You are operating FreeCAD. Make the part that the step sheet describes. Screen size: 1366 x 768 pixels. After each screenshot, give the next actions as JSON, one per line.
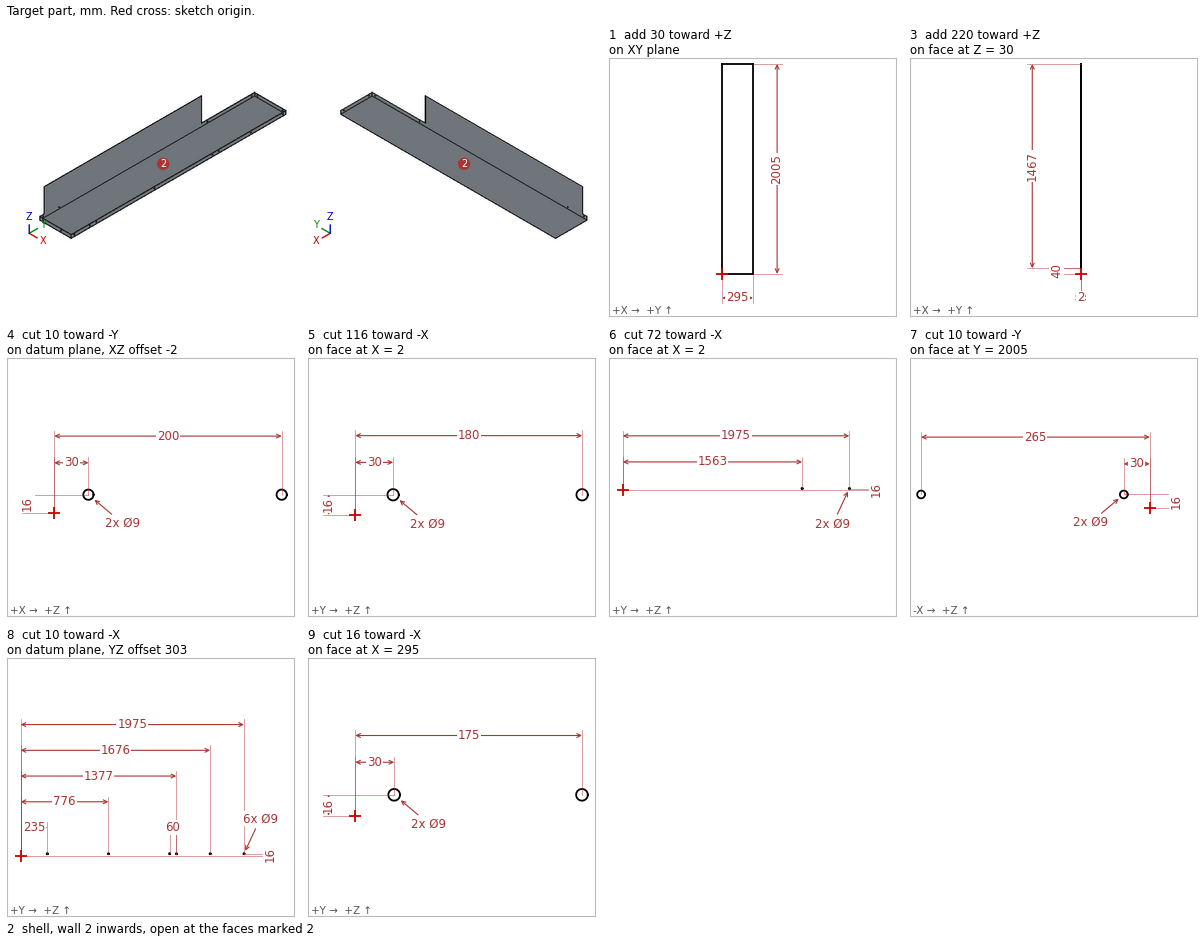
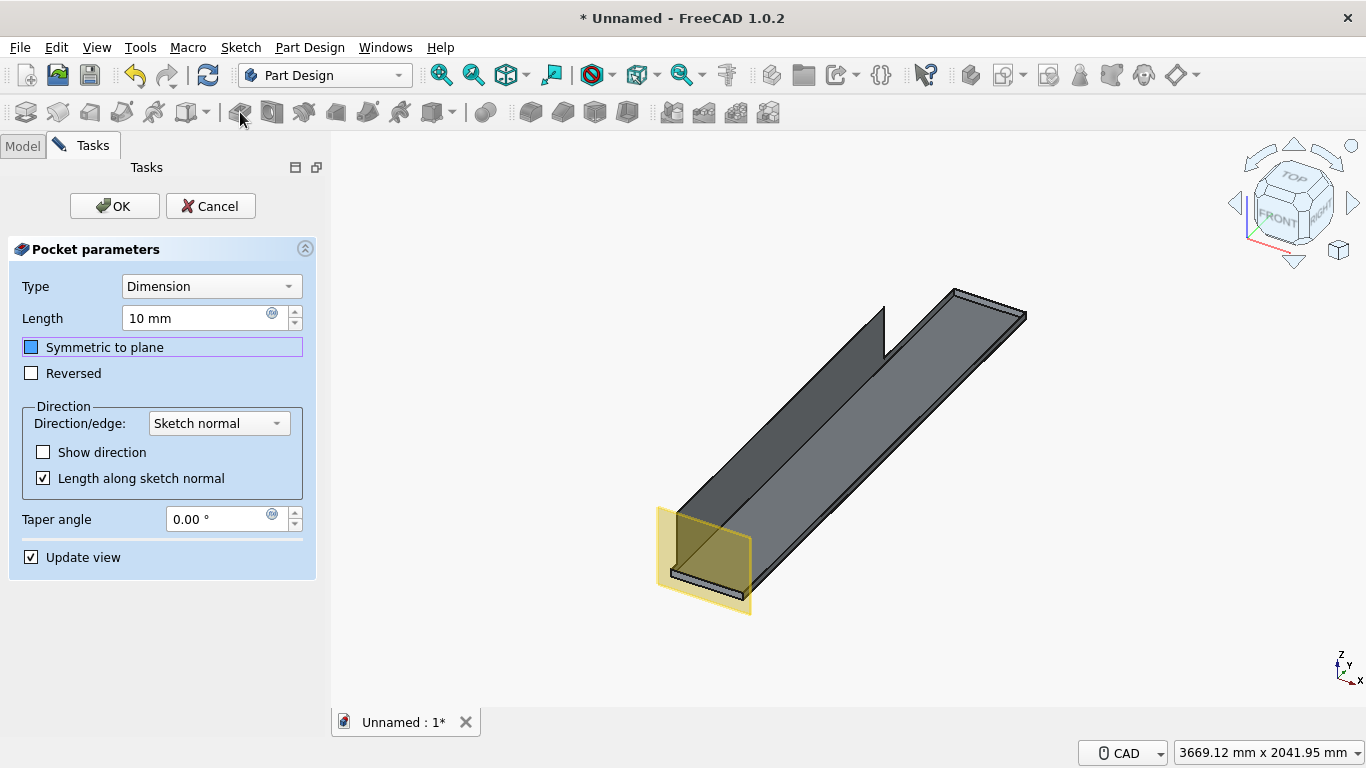
{"action": "left_click", "coordinate": [30, 373]}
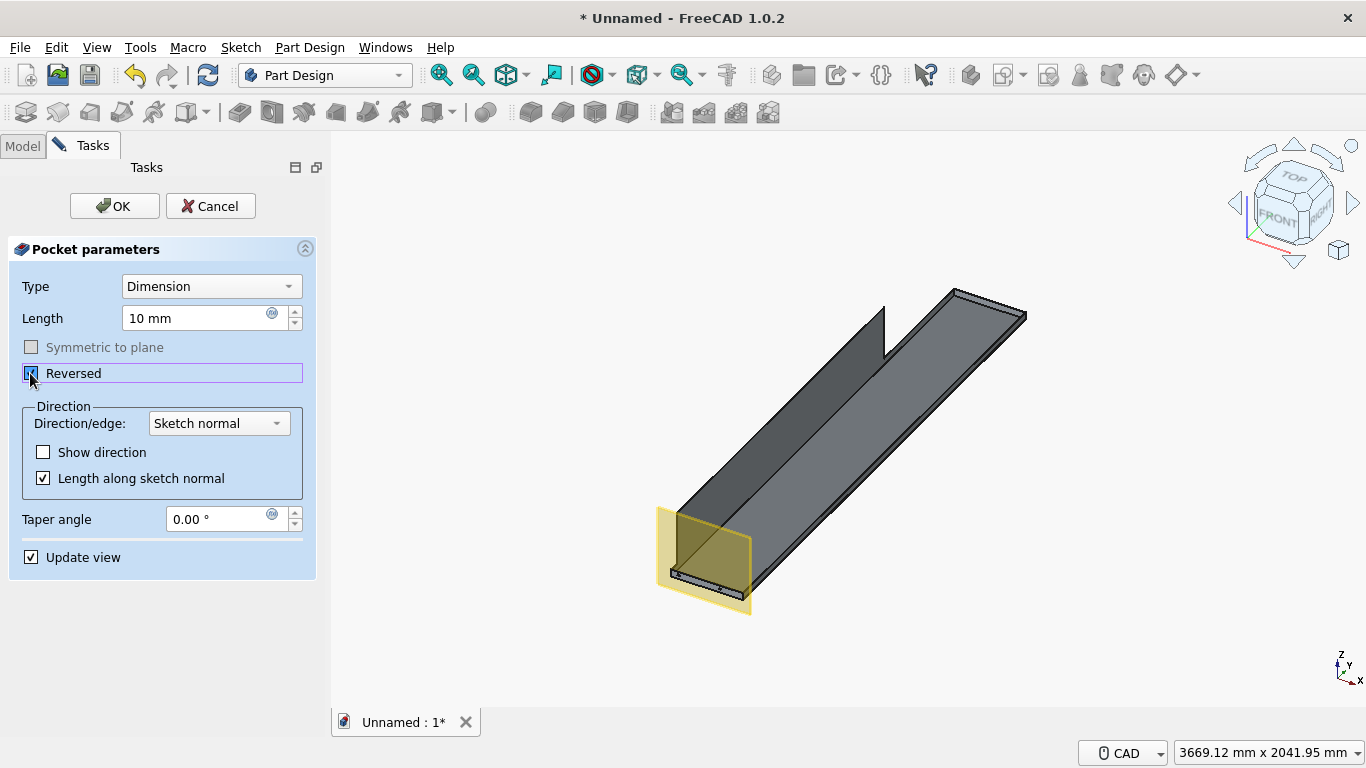
{"action": "left_click", "coordinate": [115, 206]}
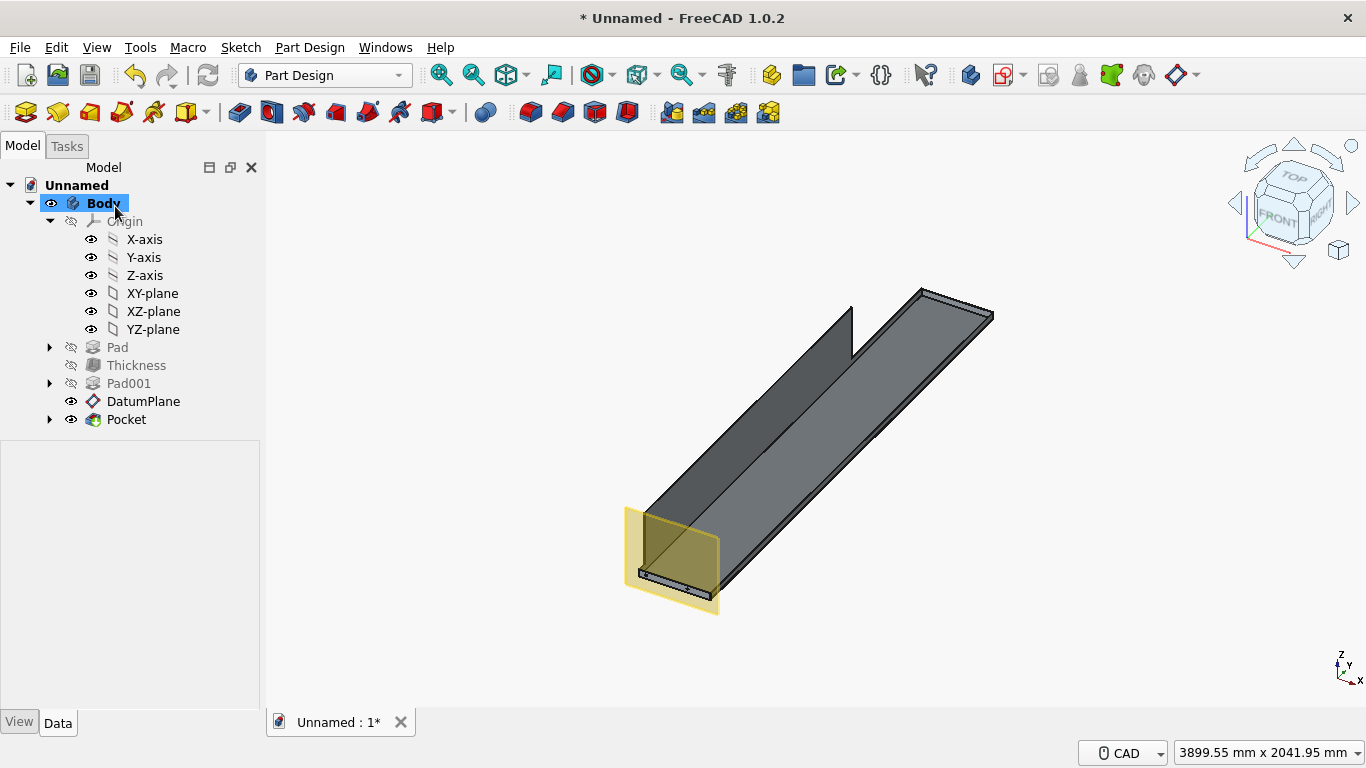
{"action": "left_click", "coordinate": [116, 401]}
{"action": "key", "text": "space"}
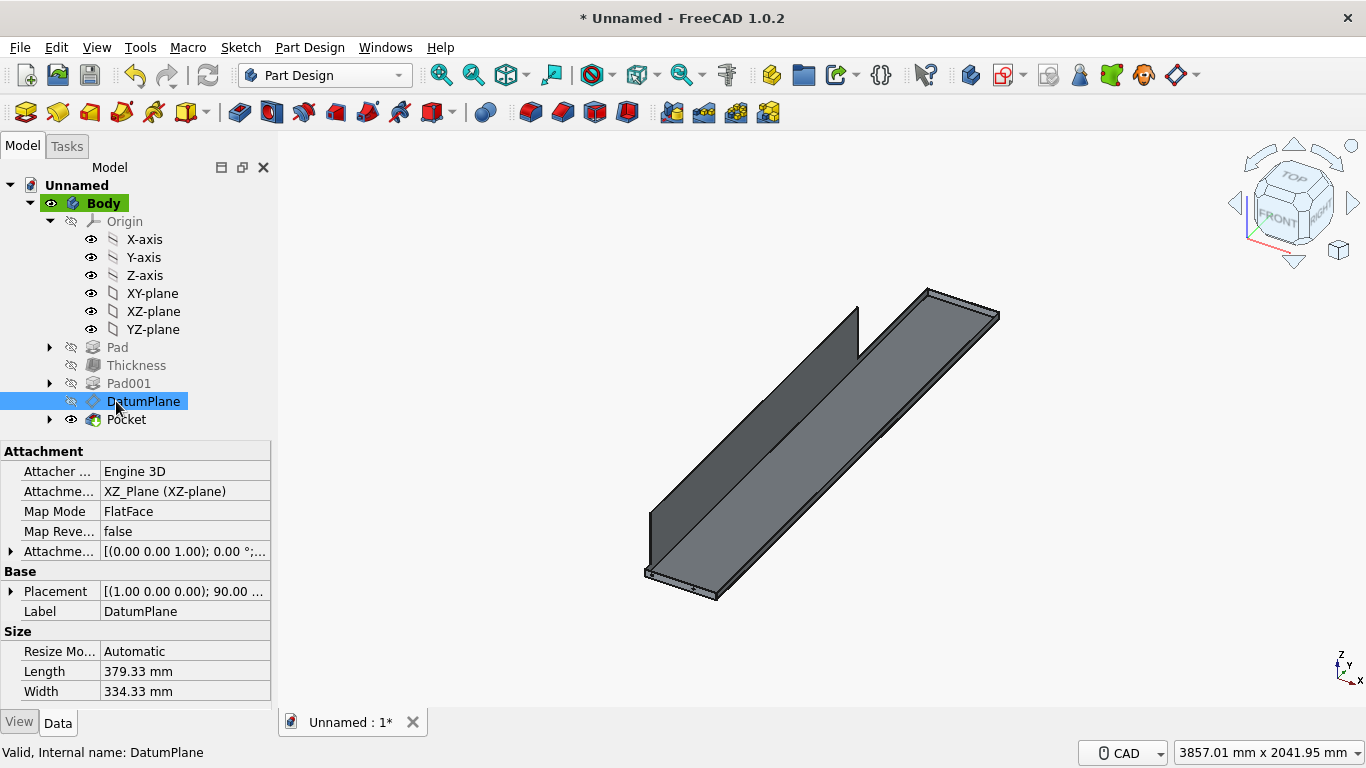
{"action": "left_click", "coordinate": [827, 366]}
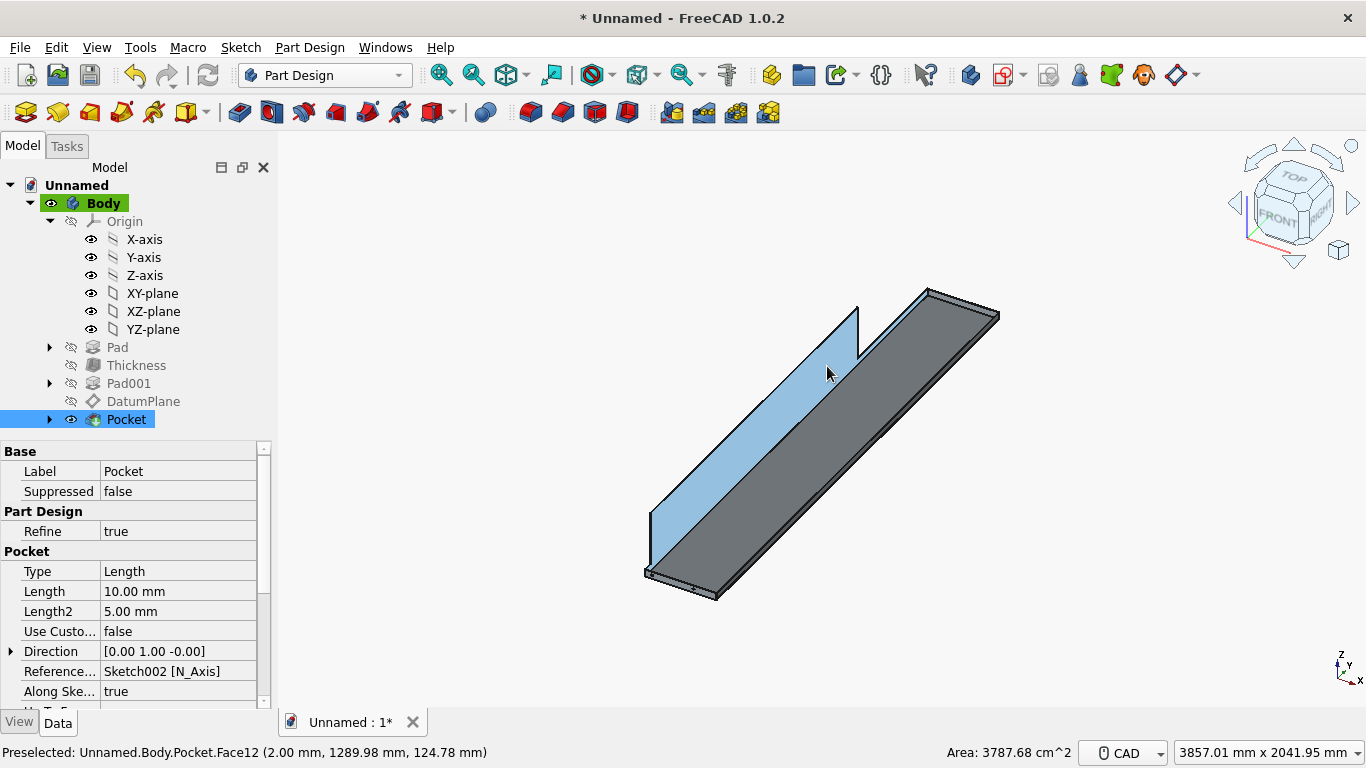
{"action": "left_click", "coordinate": [1004, 76]}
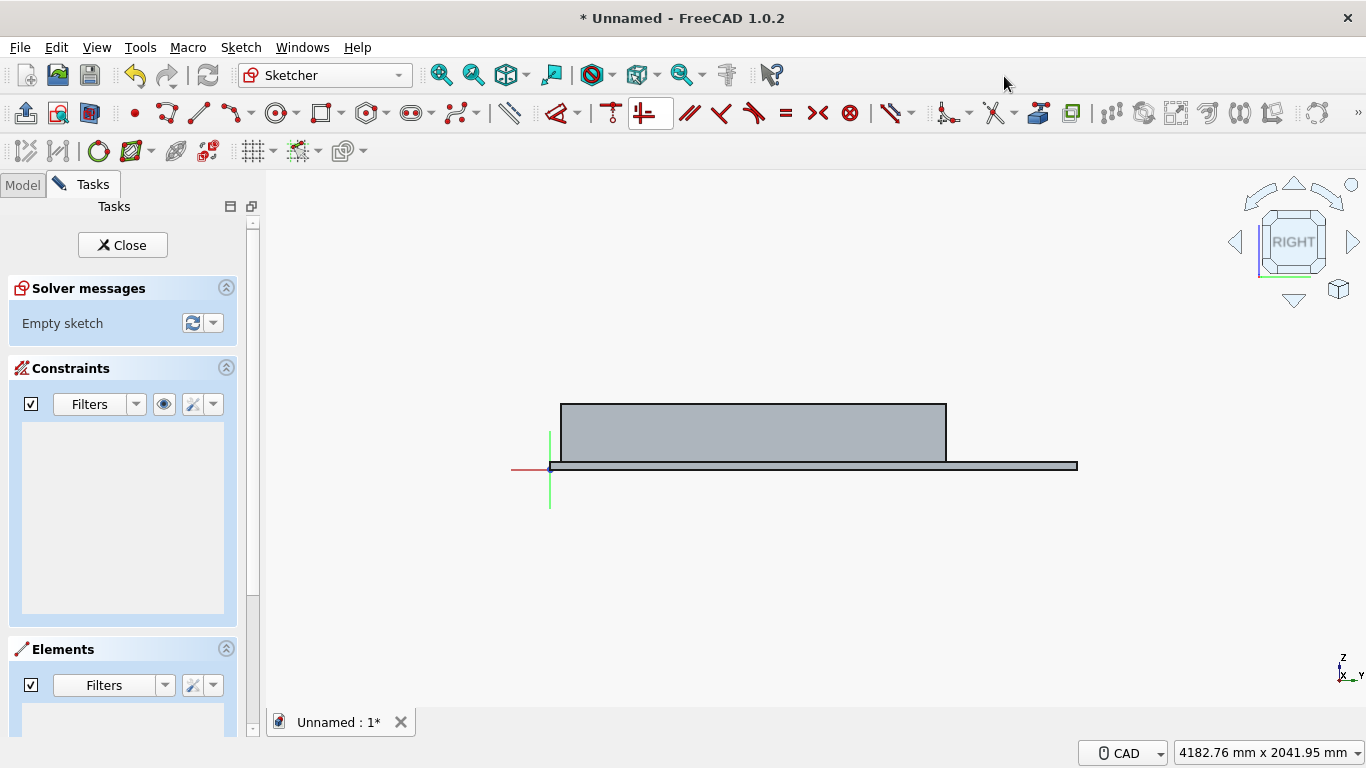
{"action": "scroll", "coordinate": [560, 469], "scroll_direction": "up", "scroll_amount": 13}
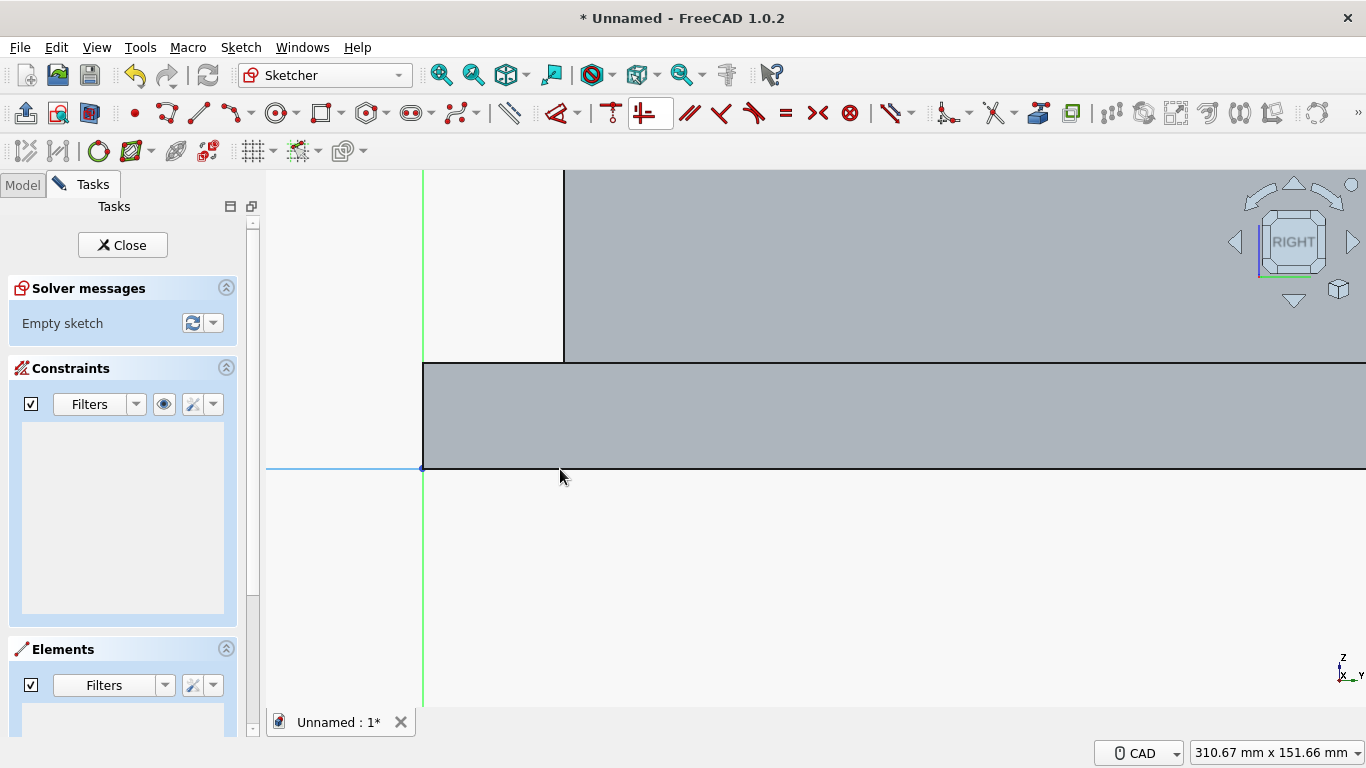
{"action": "key", "text": "g c"}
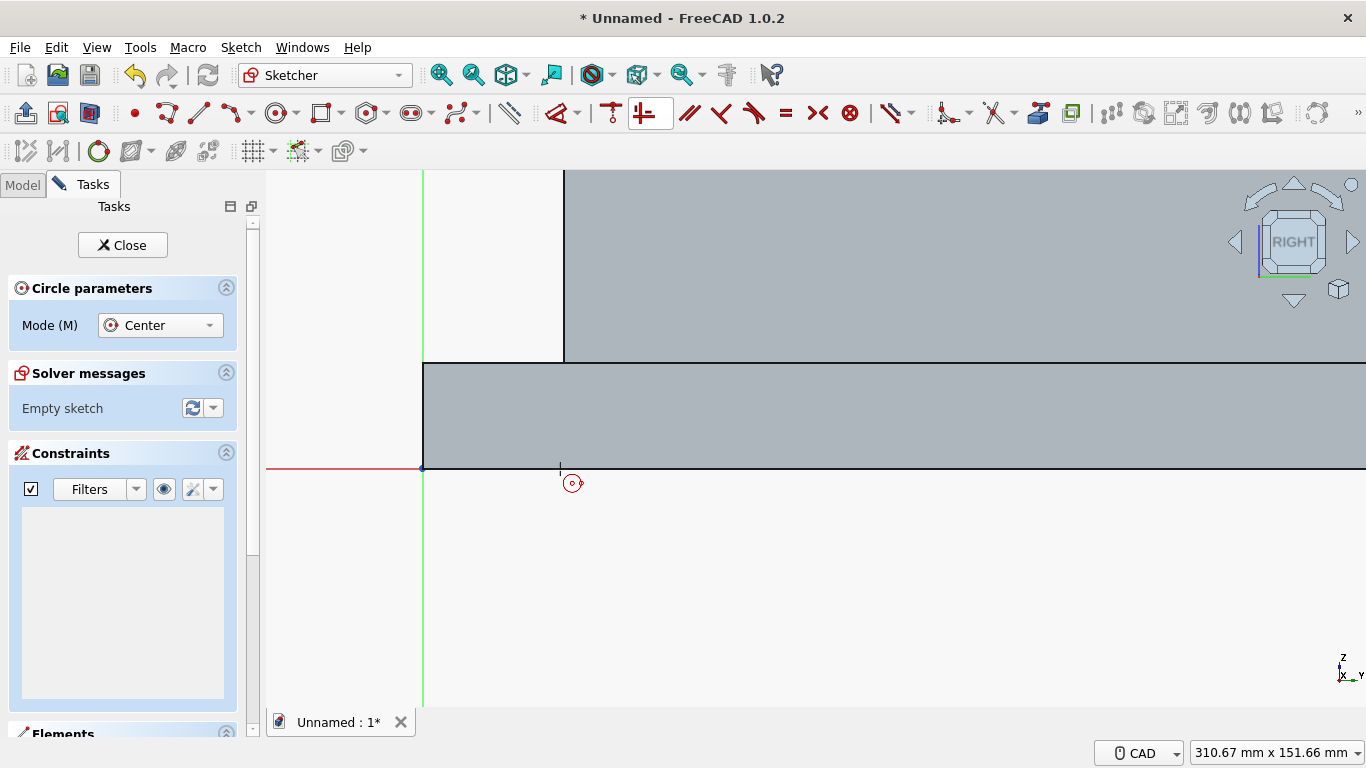
{"action": "scroll", "coordinate": [529, 412], "scroll_direction": "up", "scroll_amount": 2}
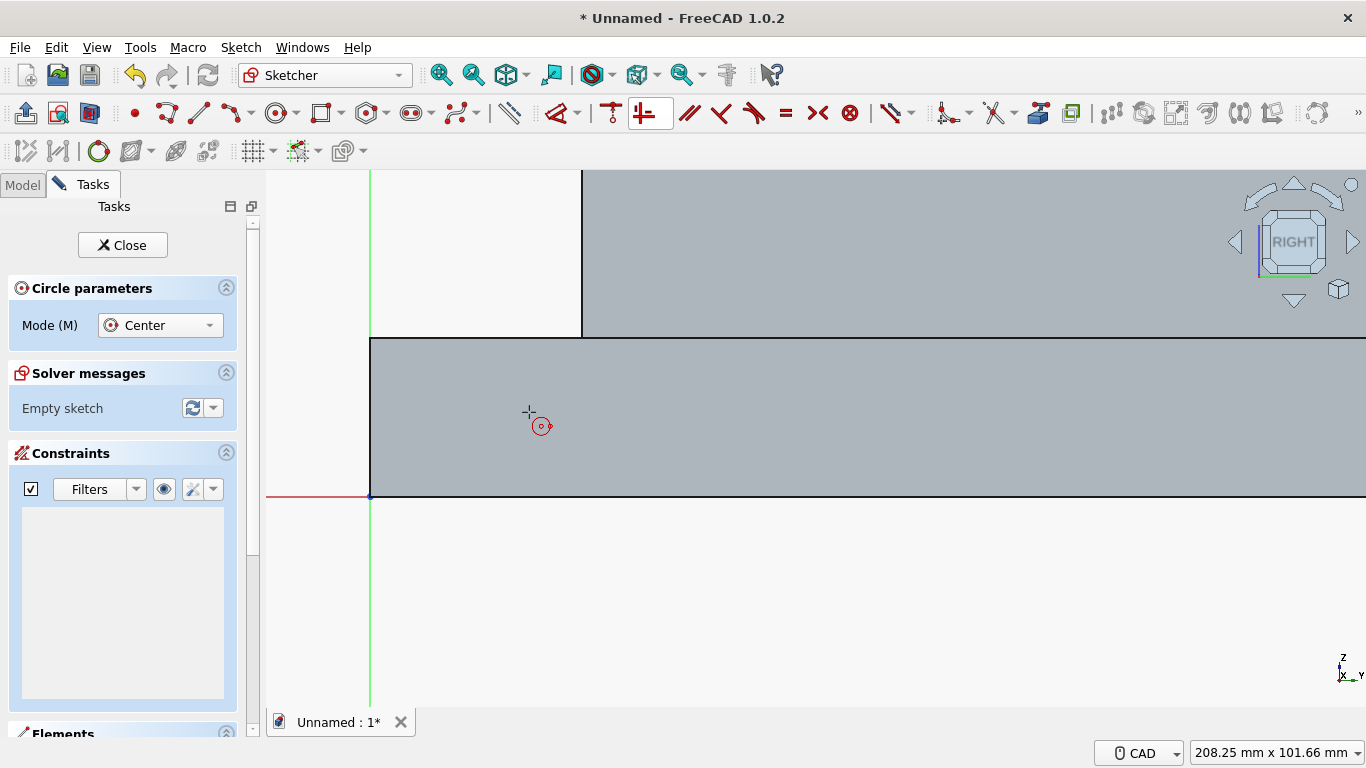
{"action": "left_click", "coordinate": [529, 412]}
{"action": "left_click", "coordinate": [546, 395]}